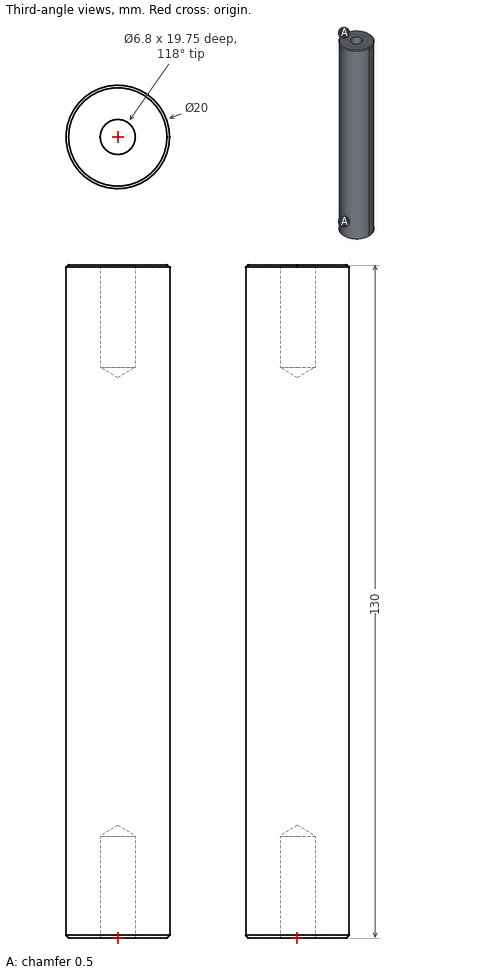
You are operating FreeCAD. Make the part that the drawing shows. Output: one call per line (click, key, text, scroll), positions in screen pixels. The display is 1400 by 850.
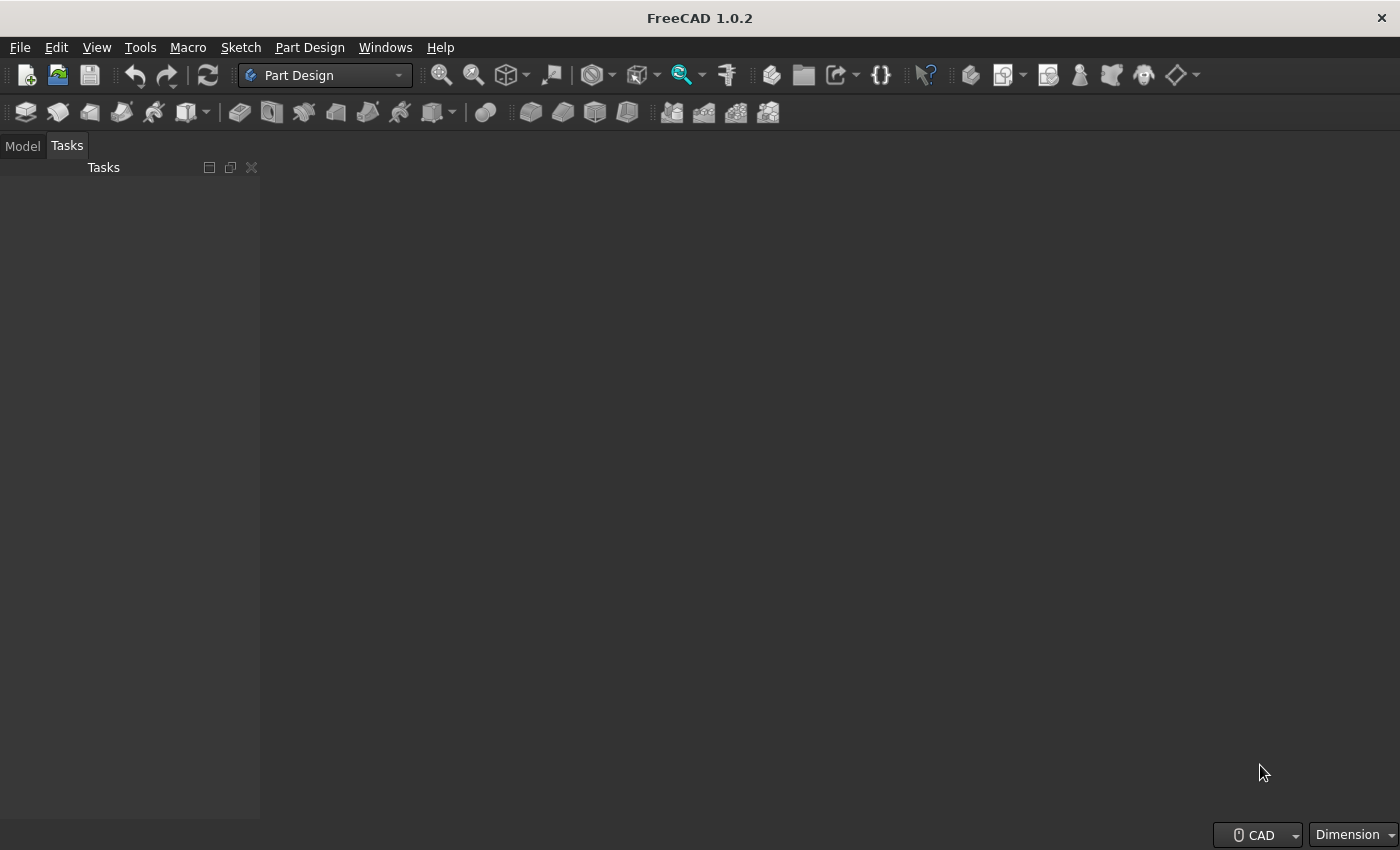
key(ctrl+n)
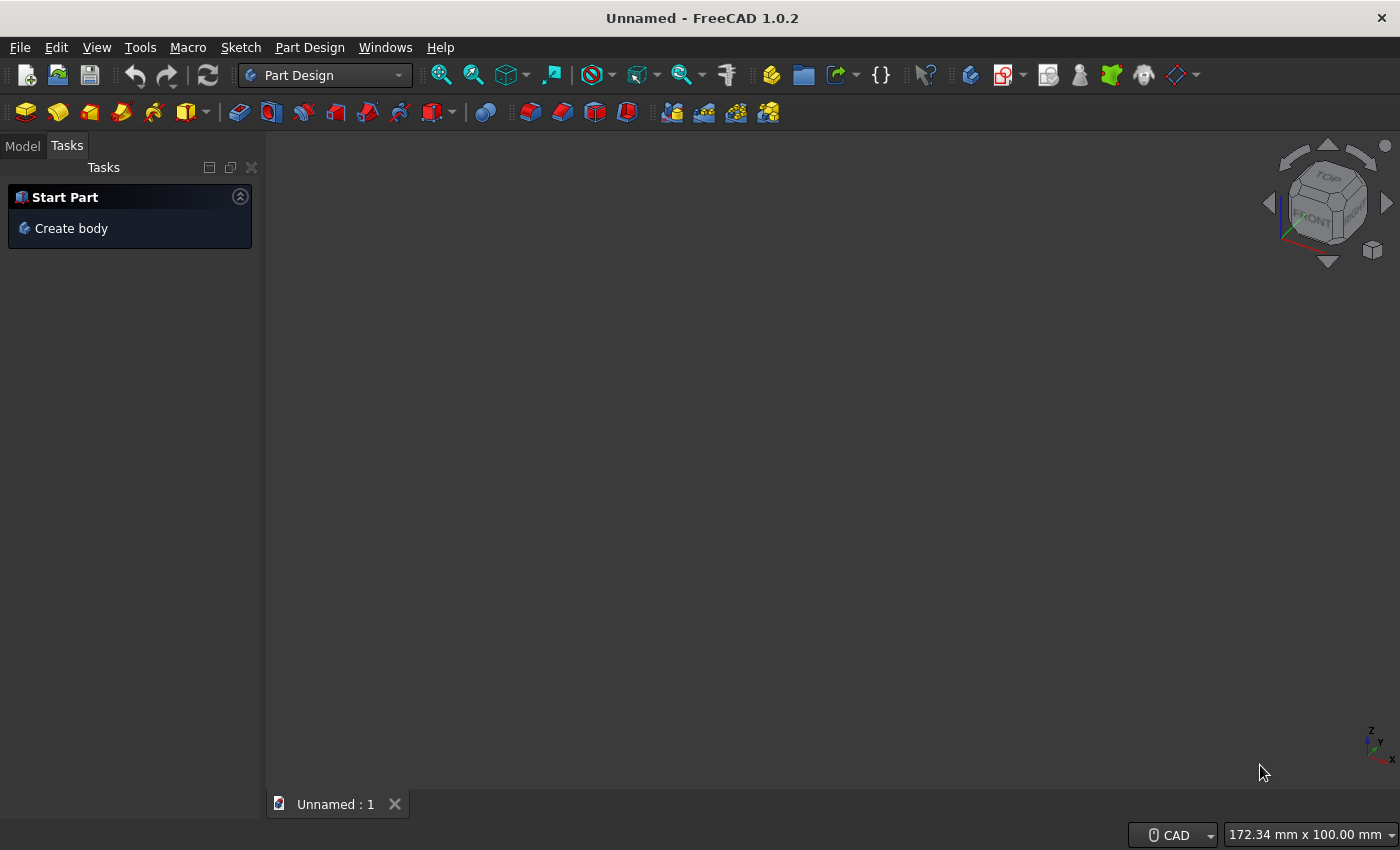
click(1004, 76)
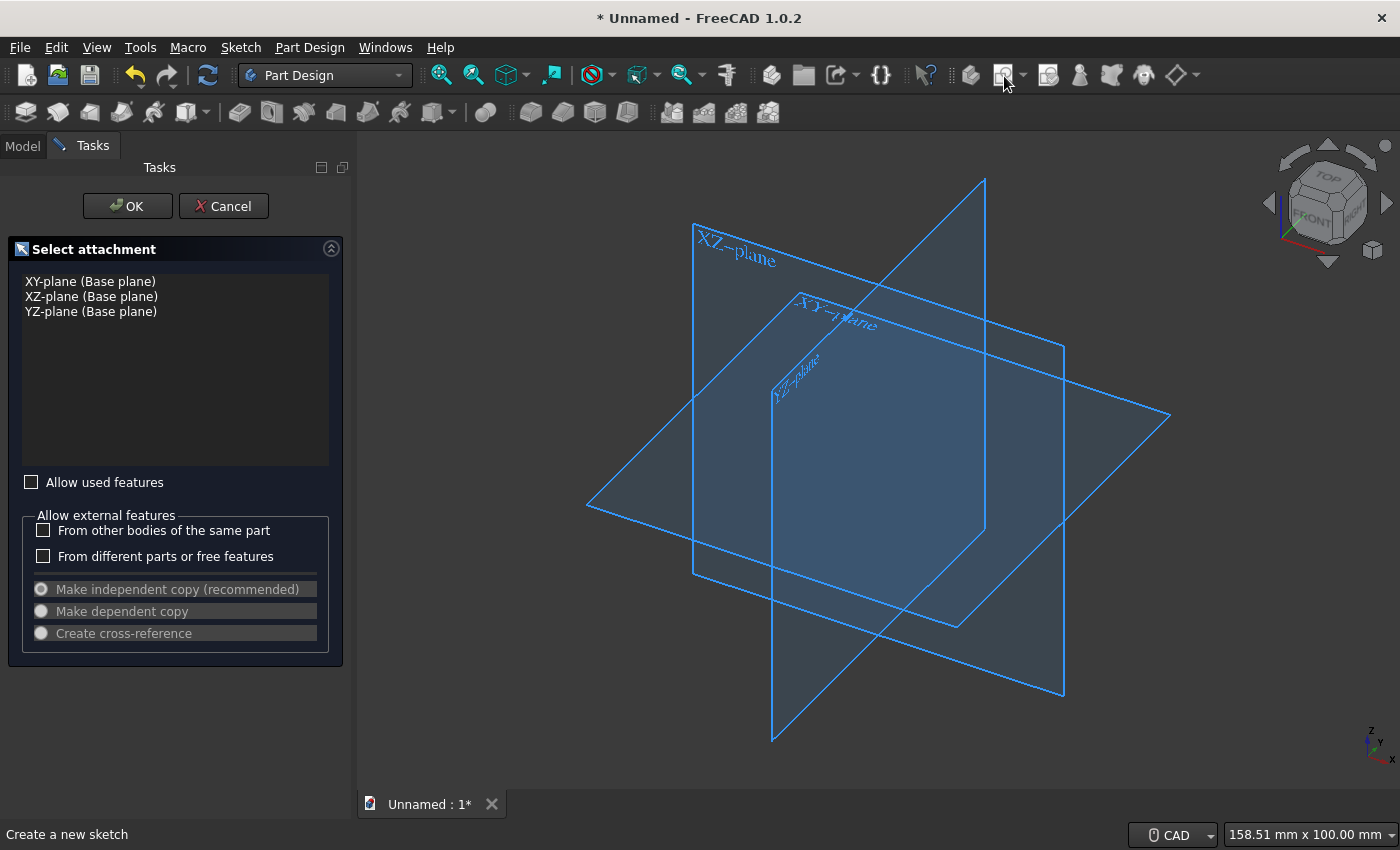
click(82, 282)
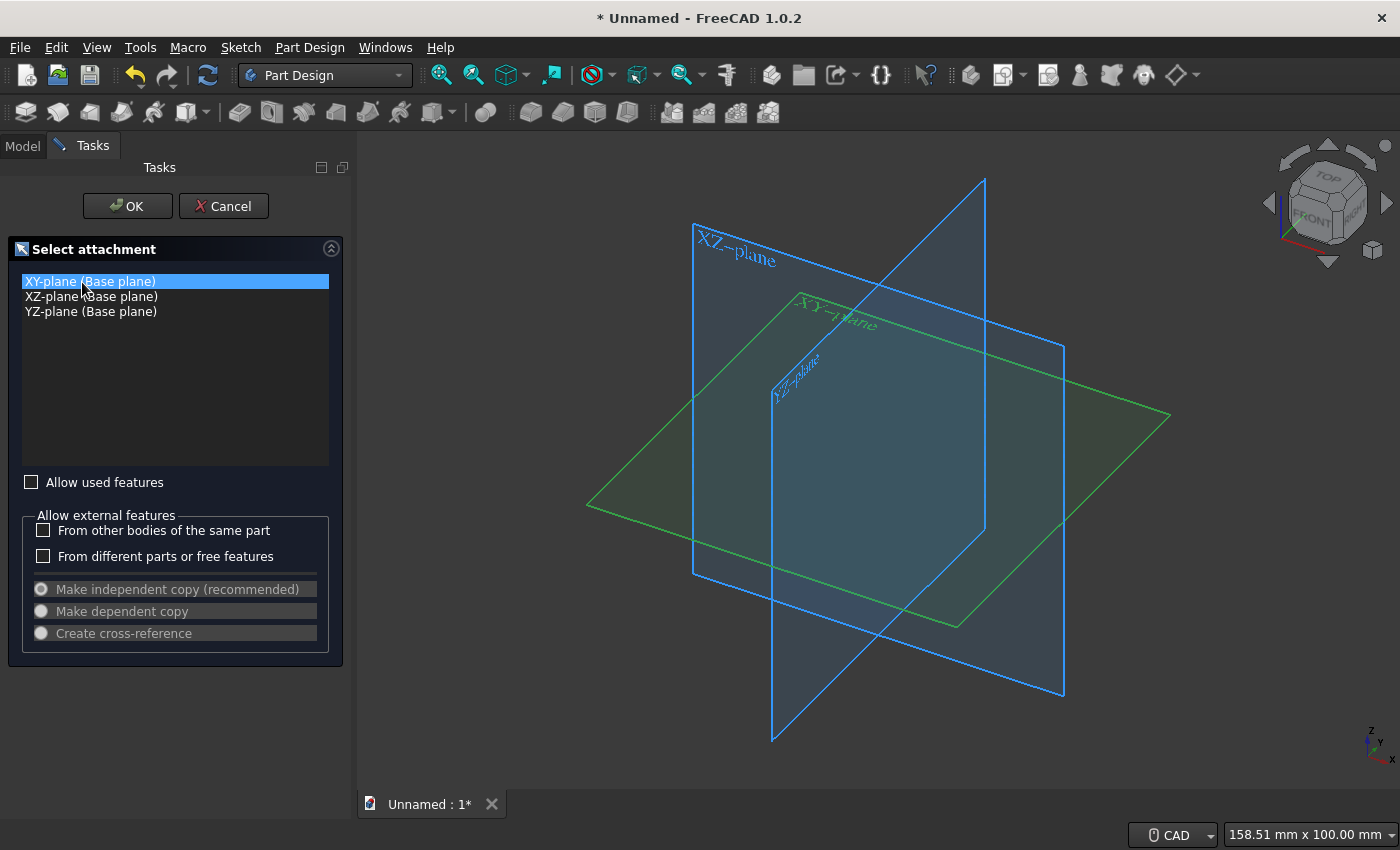
click(128, 206)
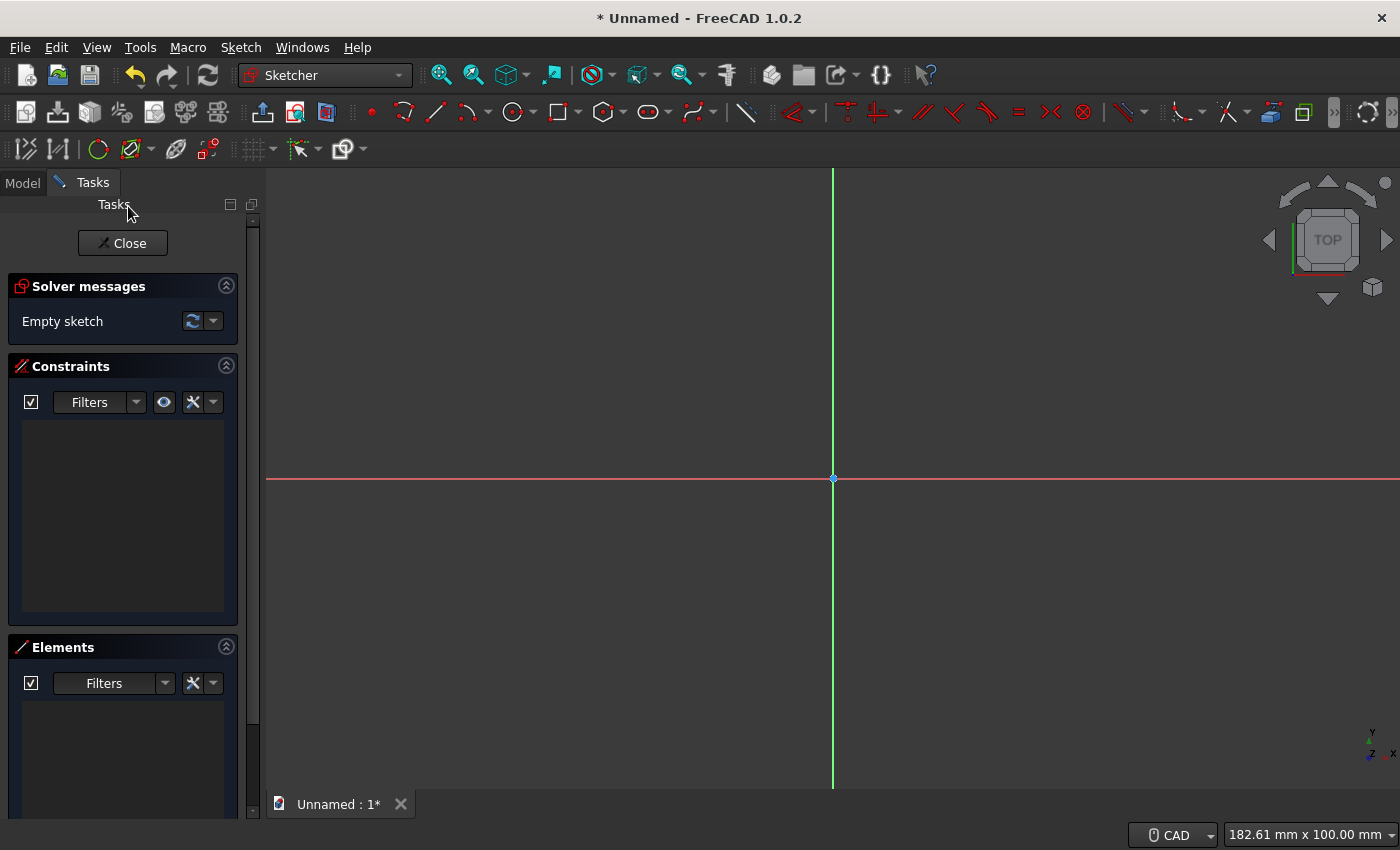
scroll(863, 478, up, 6)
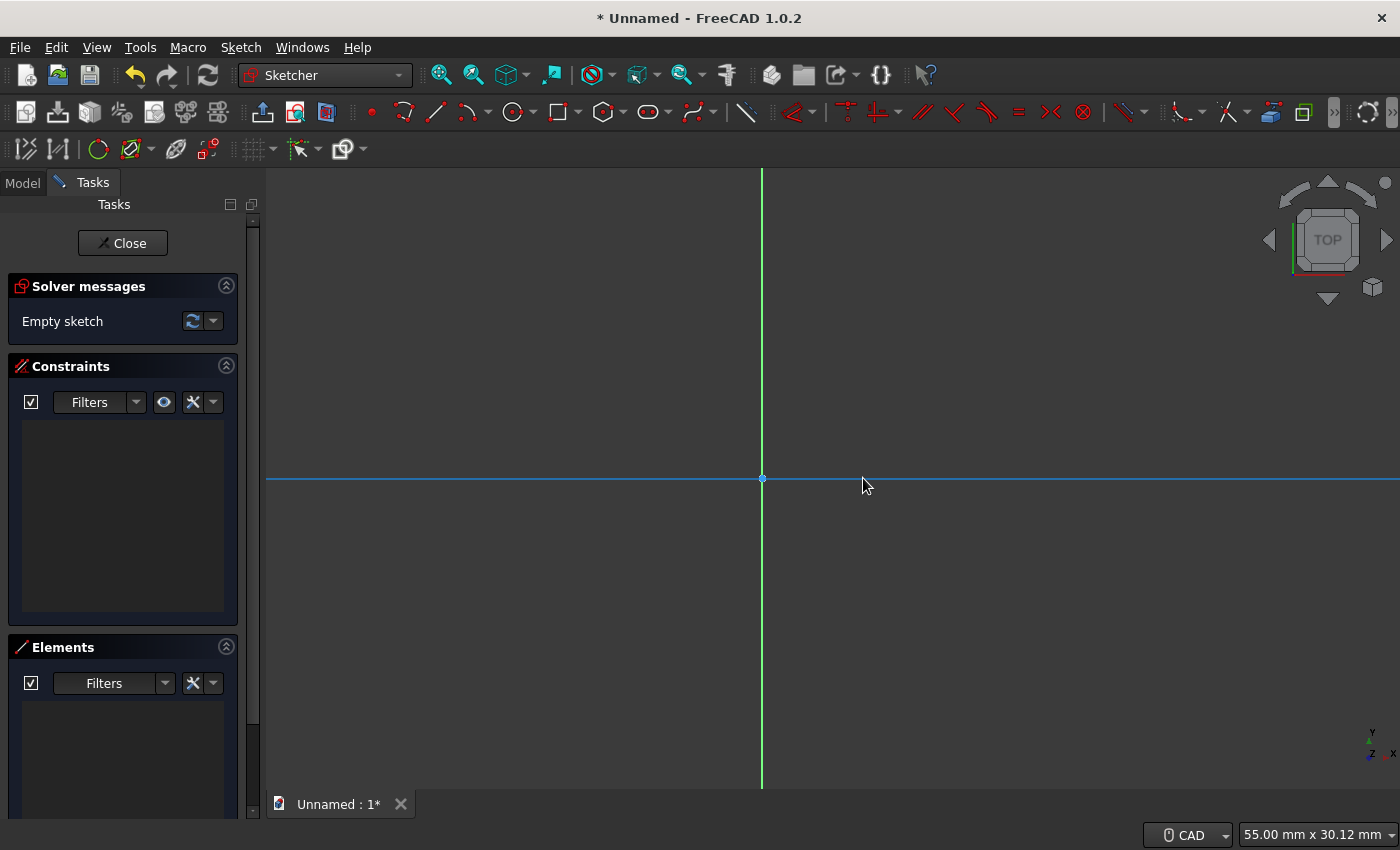
key(g)
key(c)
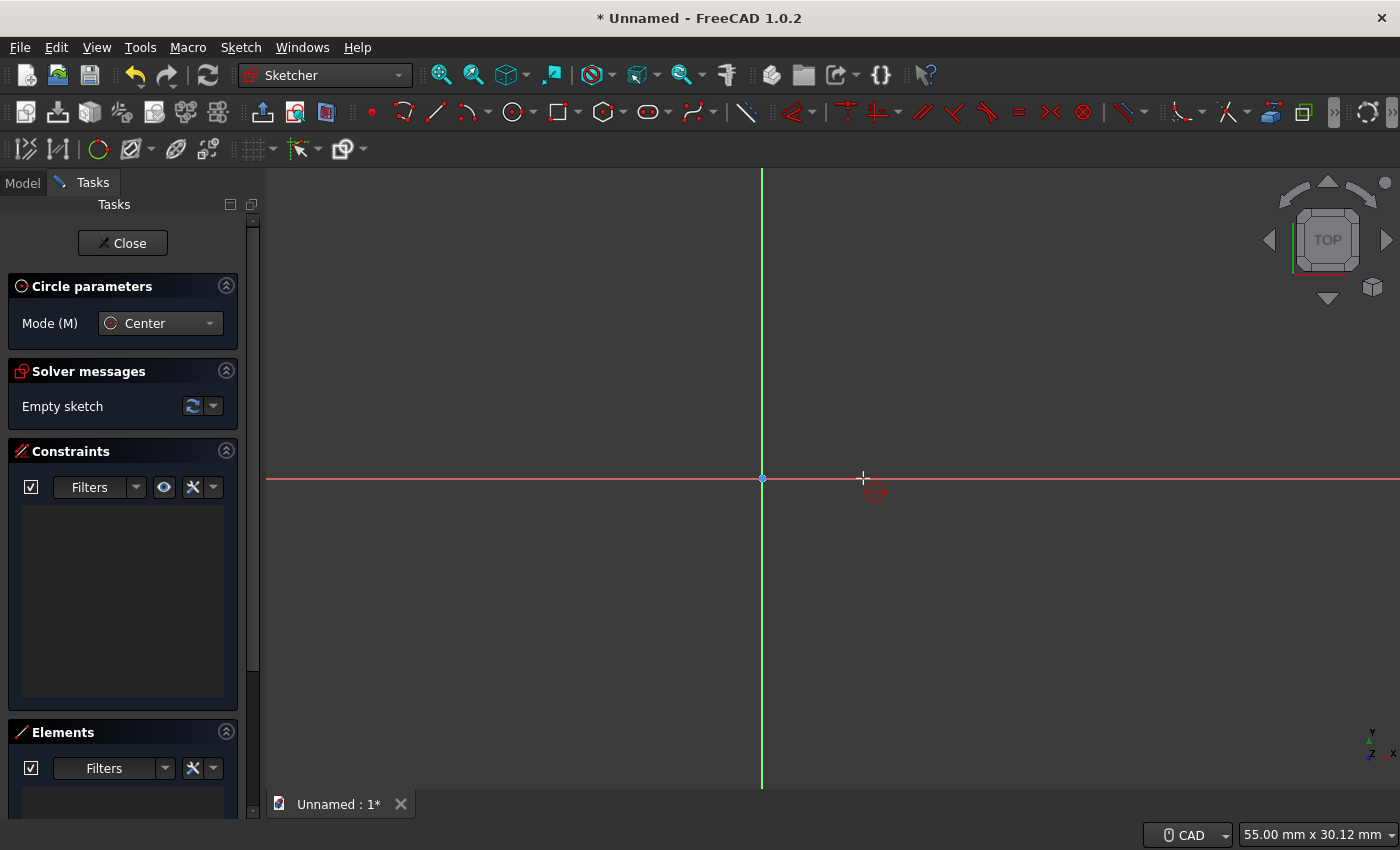
click(762, 478)
click(908, 333)
key(Escape)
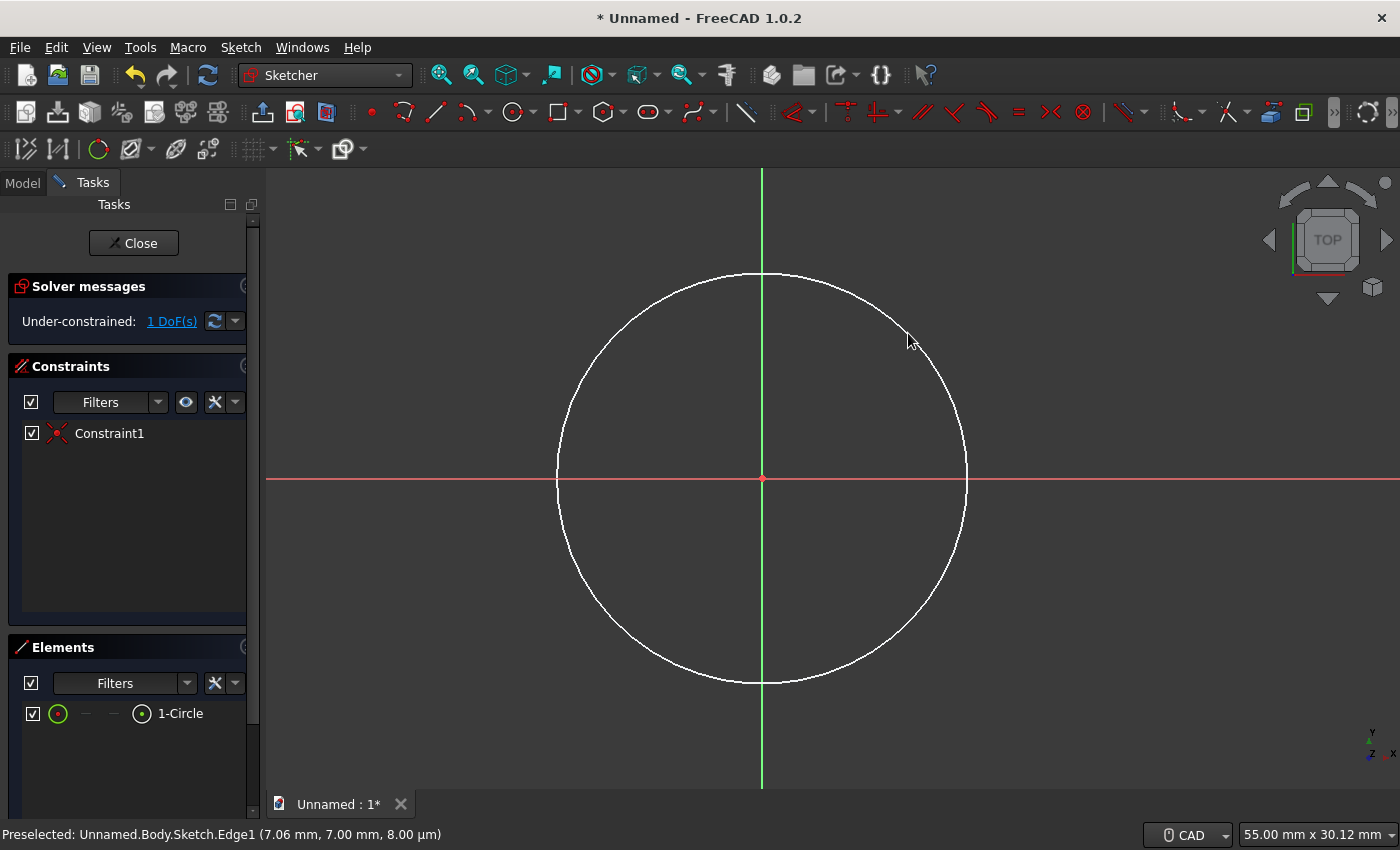
click(792, 112)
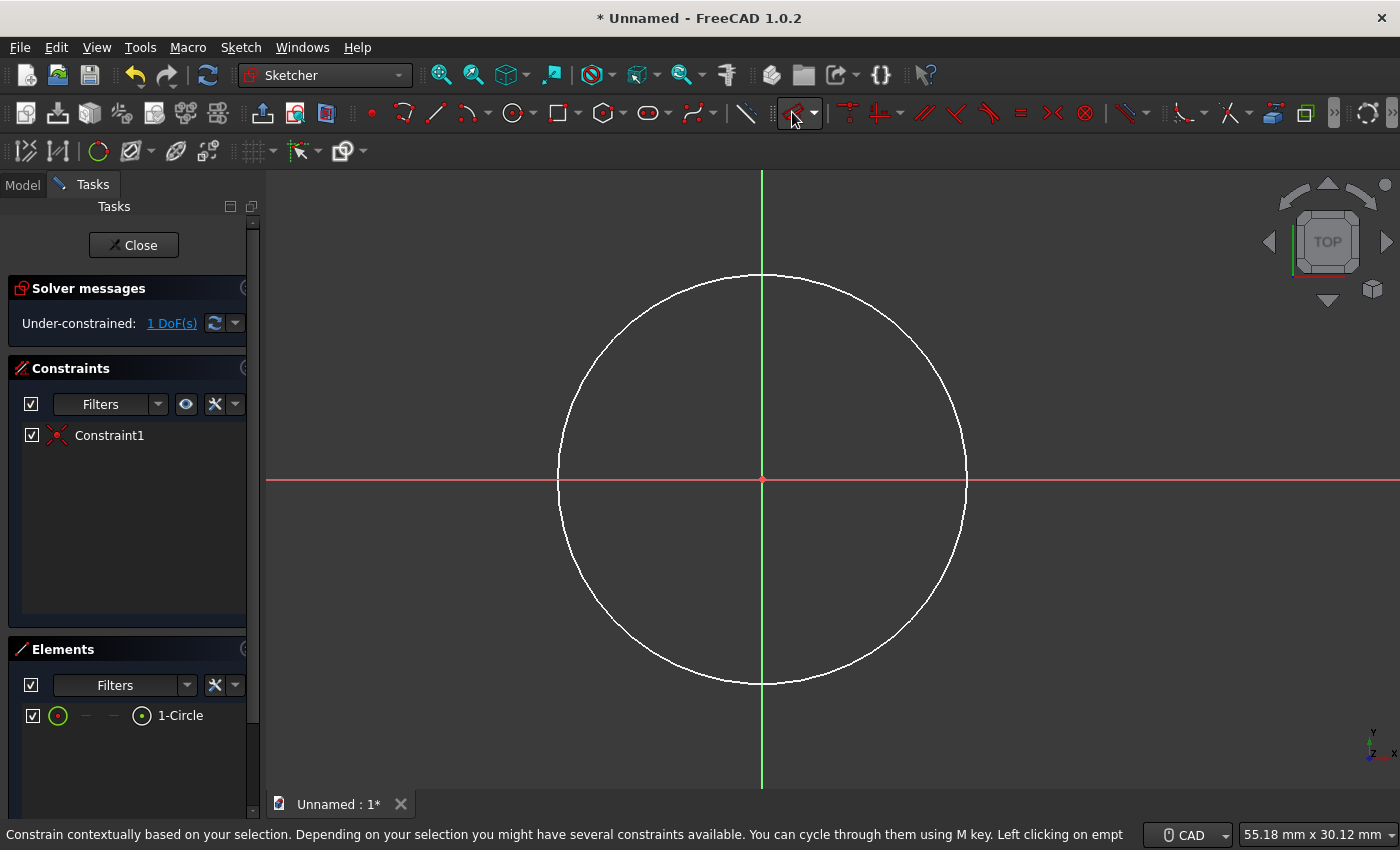
click(907, 334)
click(930, 311)